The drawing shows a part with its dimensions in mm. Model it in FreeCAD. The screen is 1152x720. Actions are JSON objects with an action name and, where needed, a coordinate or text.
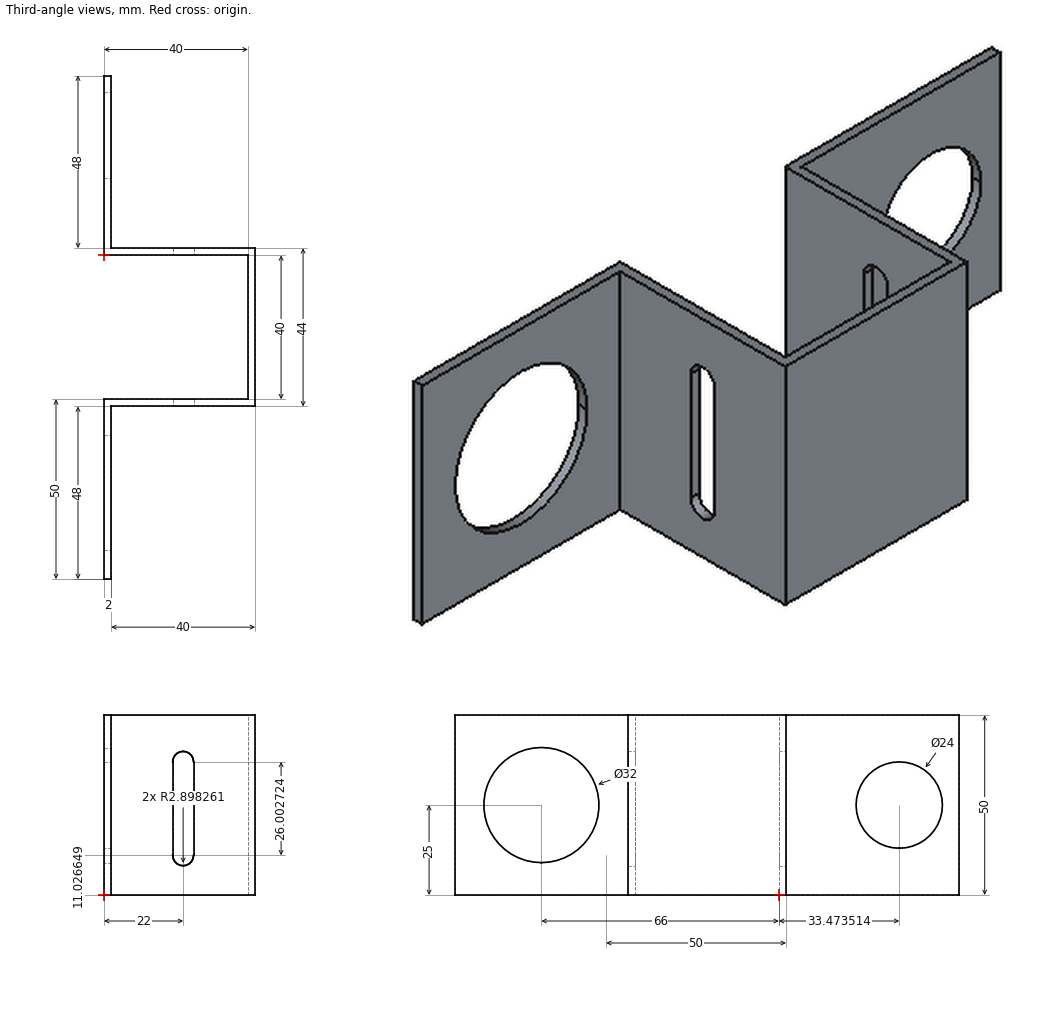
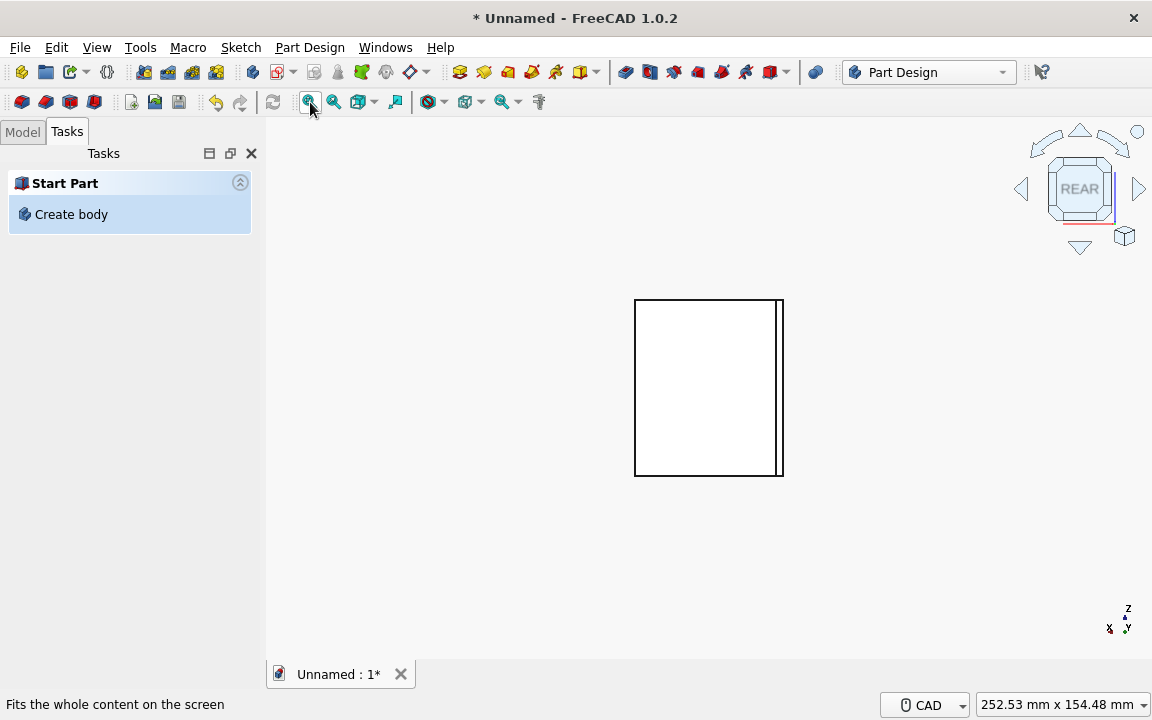
{"action": "left_click", "coordinate": [310, 102]}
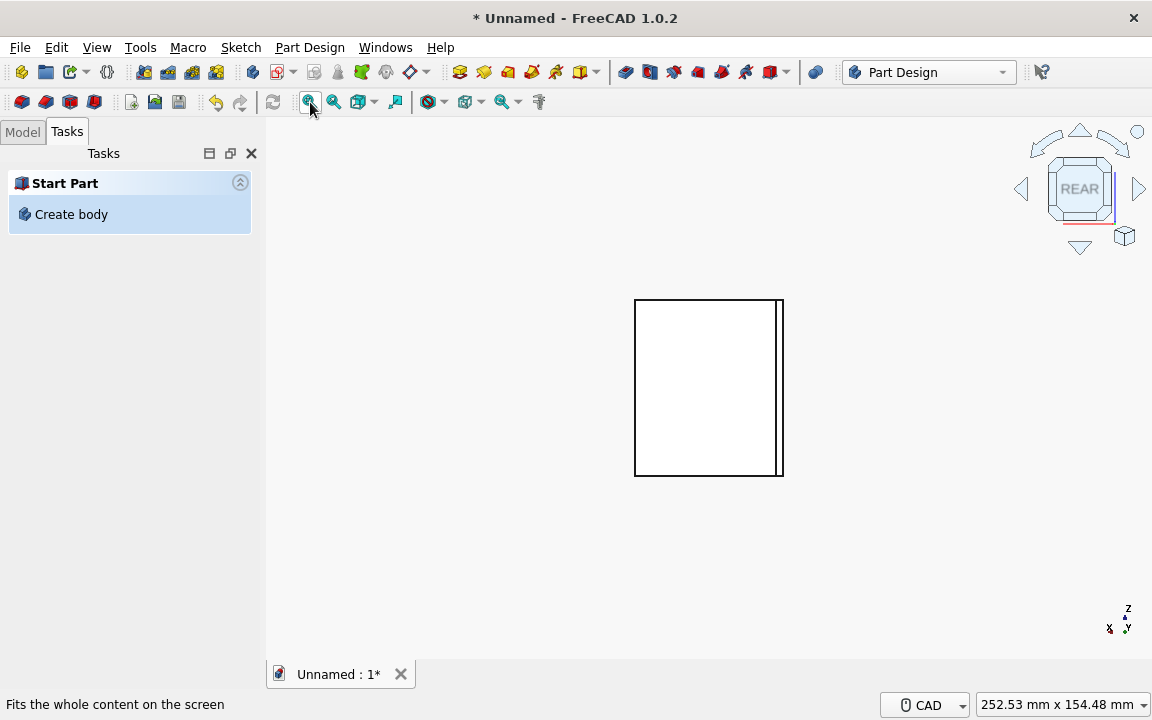
{"action": "left_click", "coordinate": [705, 387]}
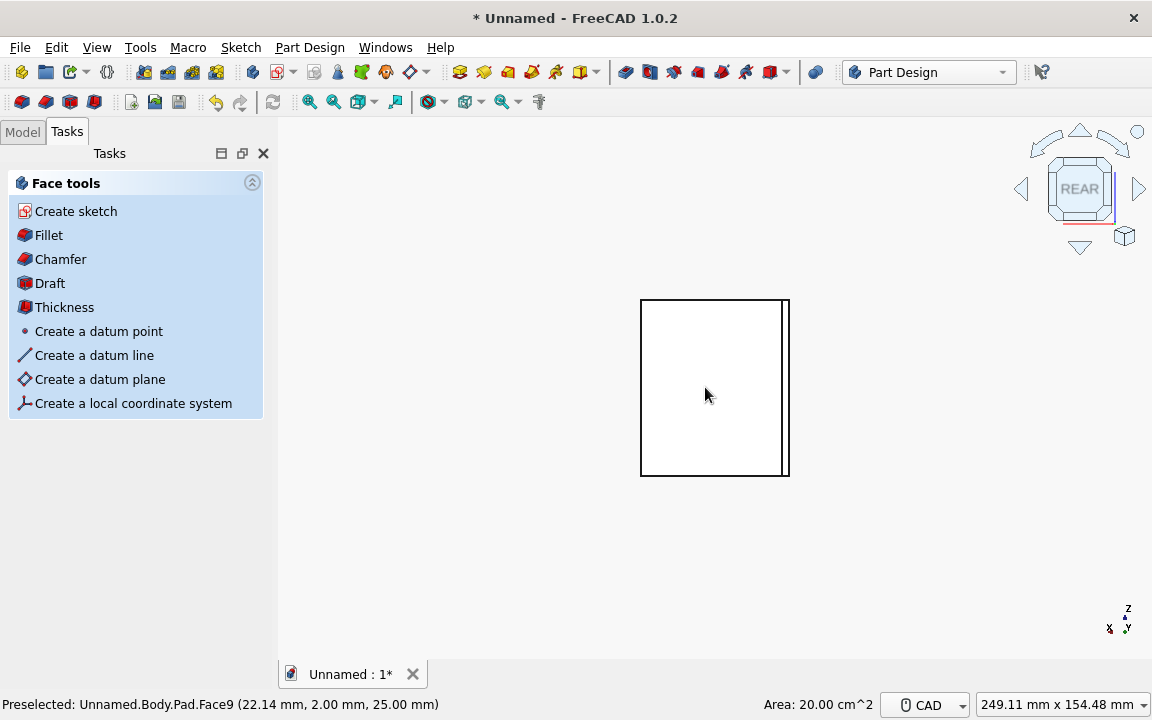
{"action": "left_click", "coordinate": [278, 72]}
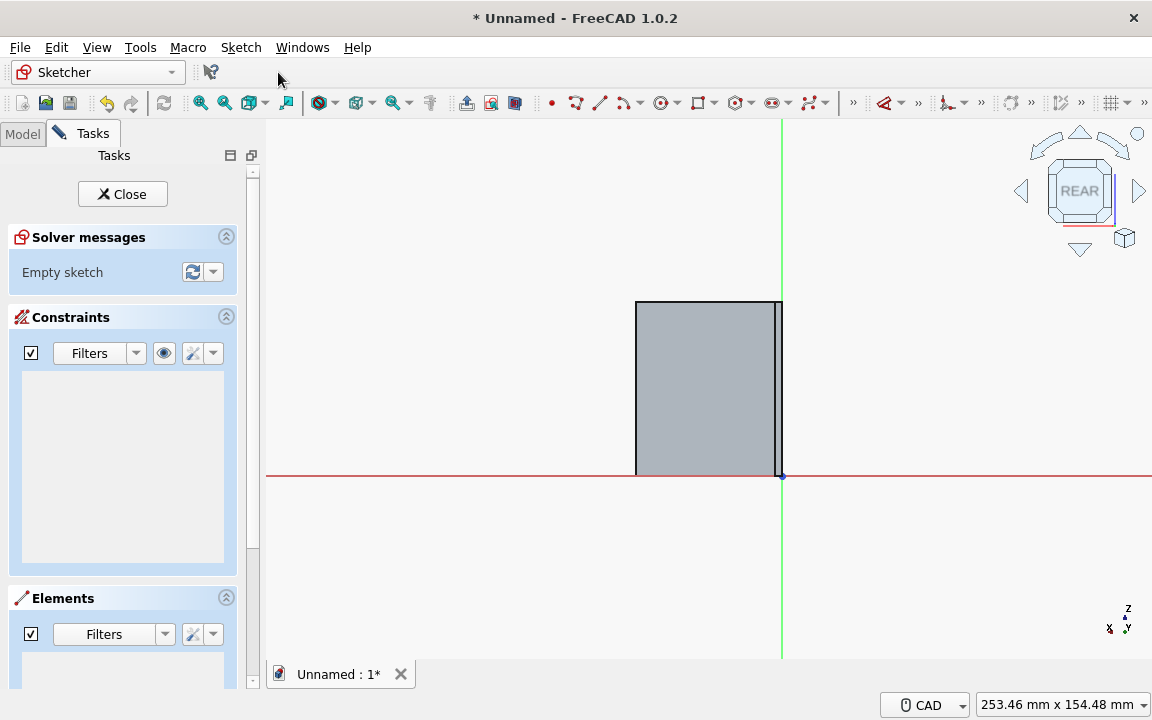
{"action": "left_click", "coordinate": [516, 104]}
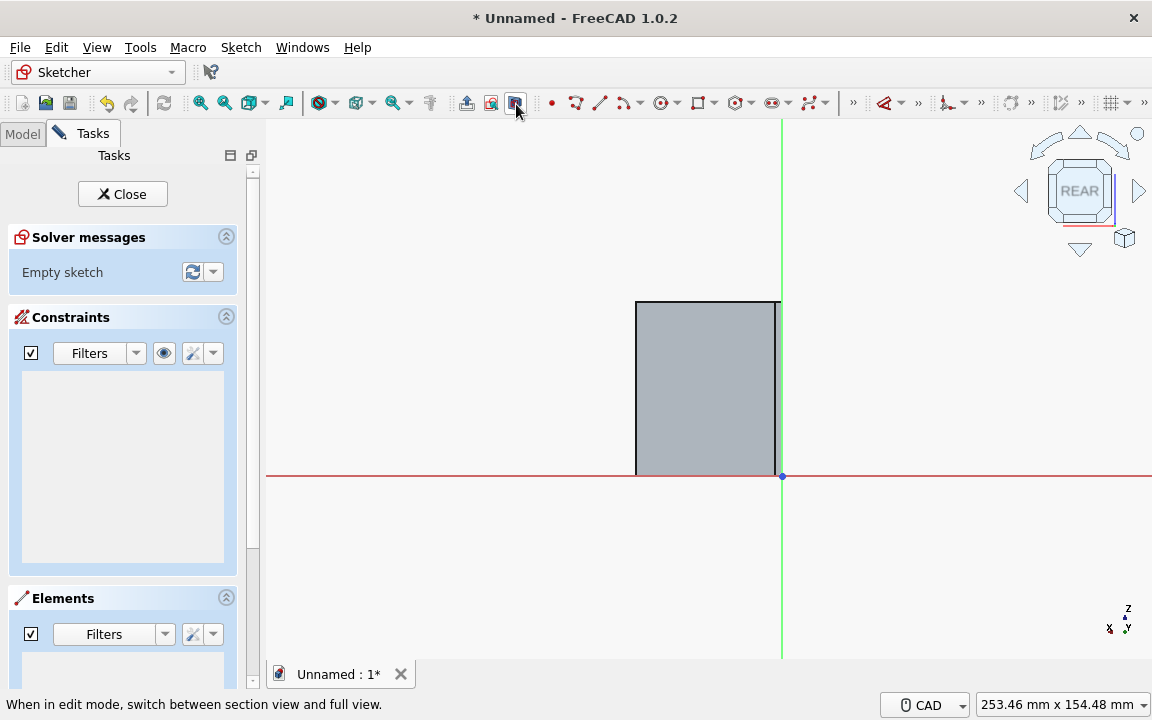
{"action": "scroll", "coordinate": [819, 421], "scroll_direction": "up", "scroll_amount": 4}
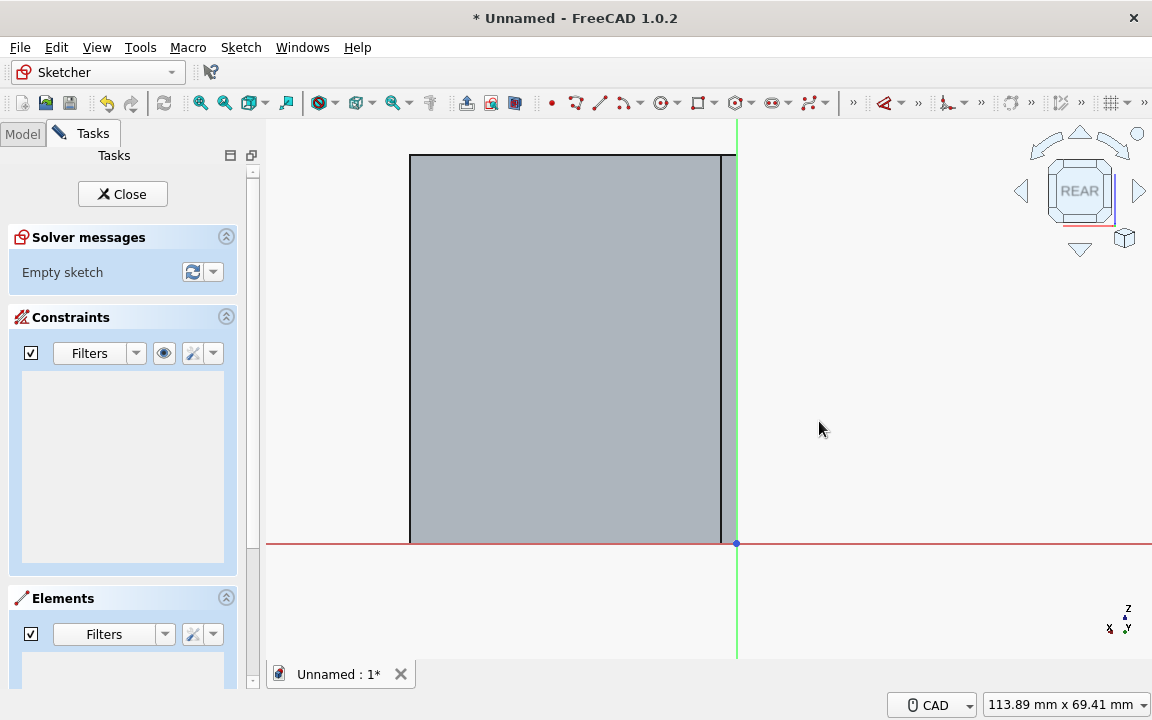
{"action": "left_click", "coordinate": [772, 104]}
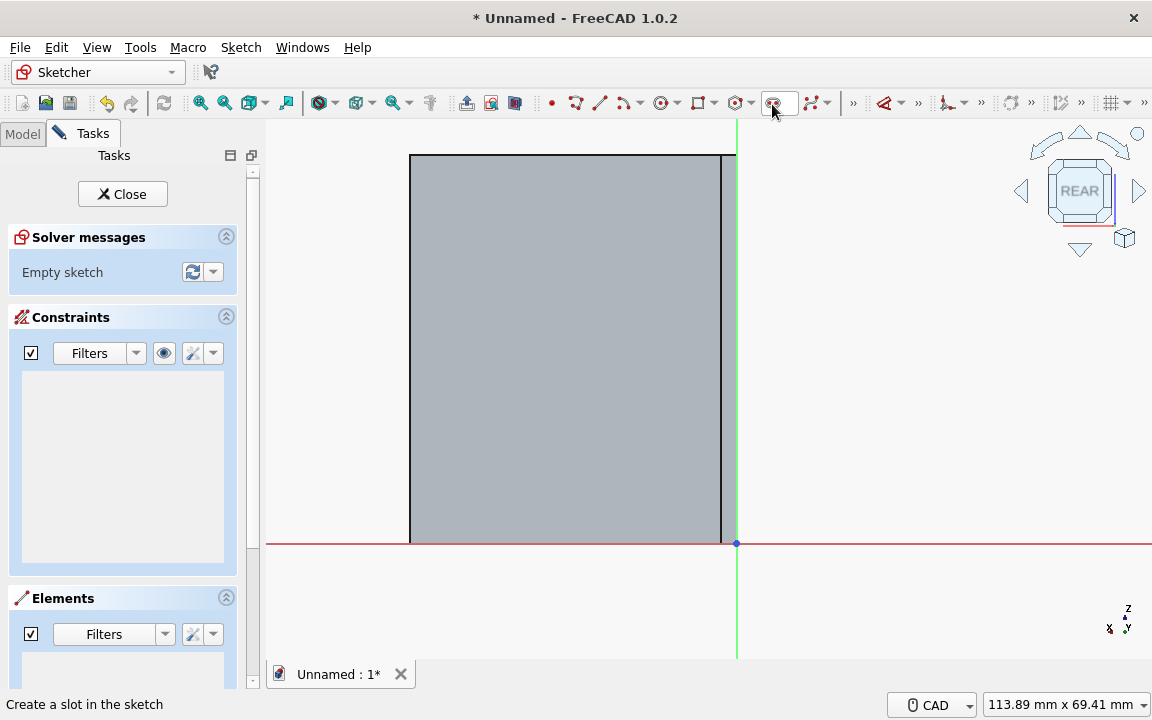
{"action": "left_click", "coordinate": [566, 458]}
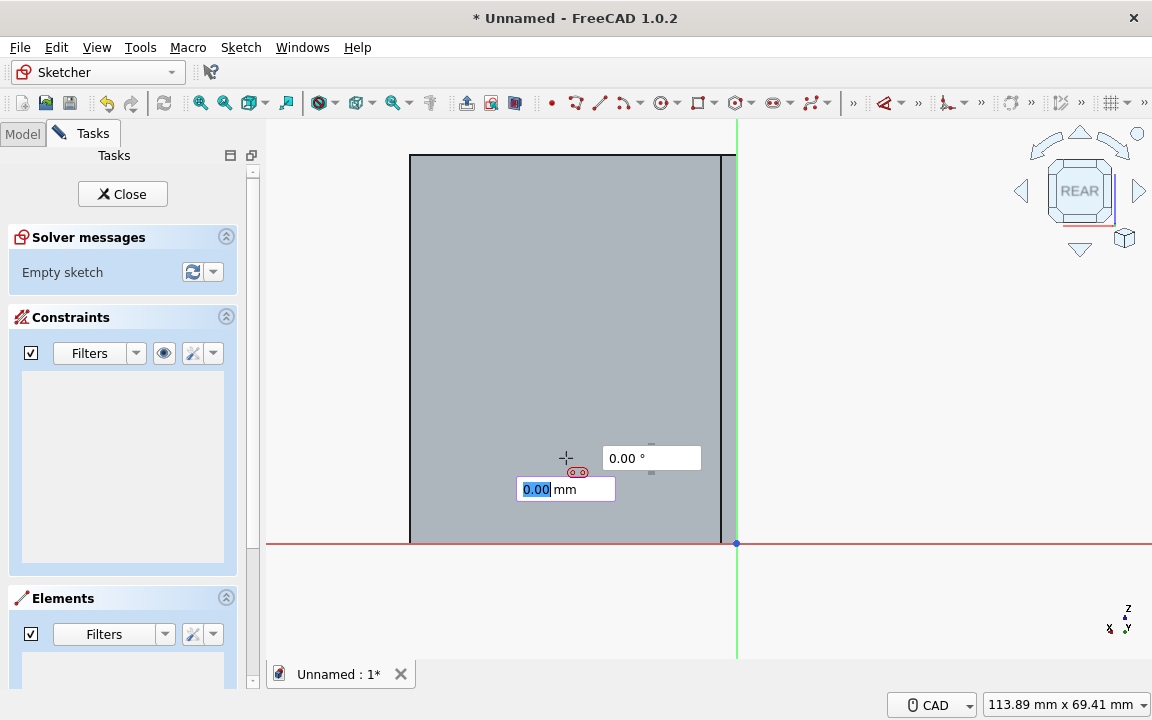
{"action": "left_click", "coordinate": [566, 256]}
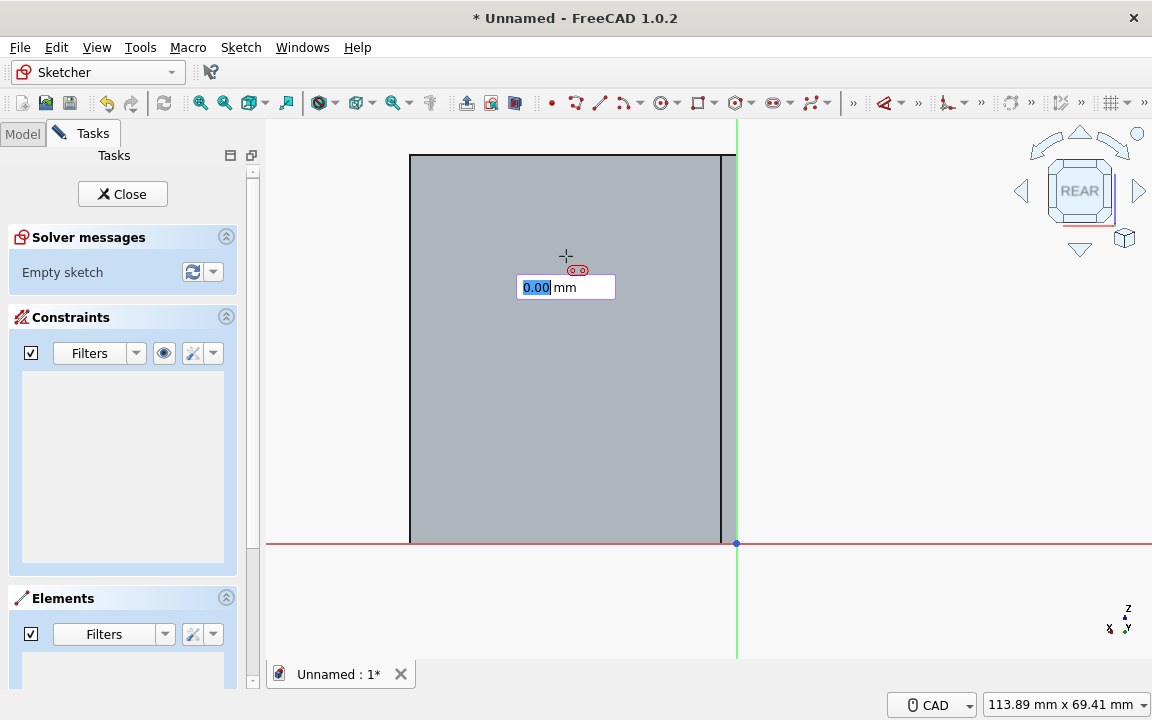
{"action": "left_click", "coordinate": [543, 357]}
{"action": "key", "text": "Escape"}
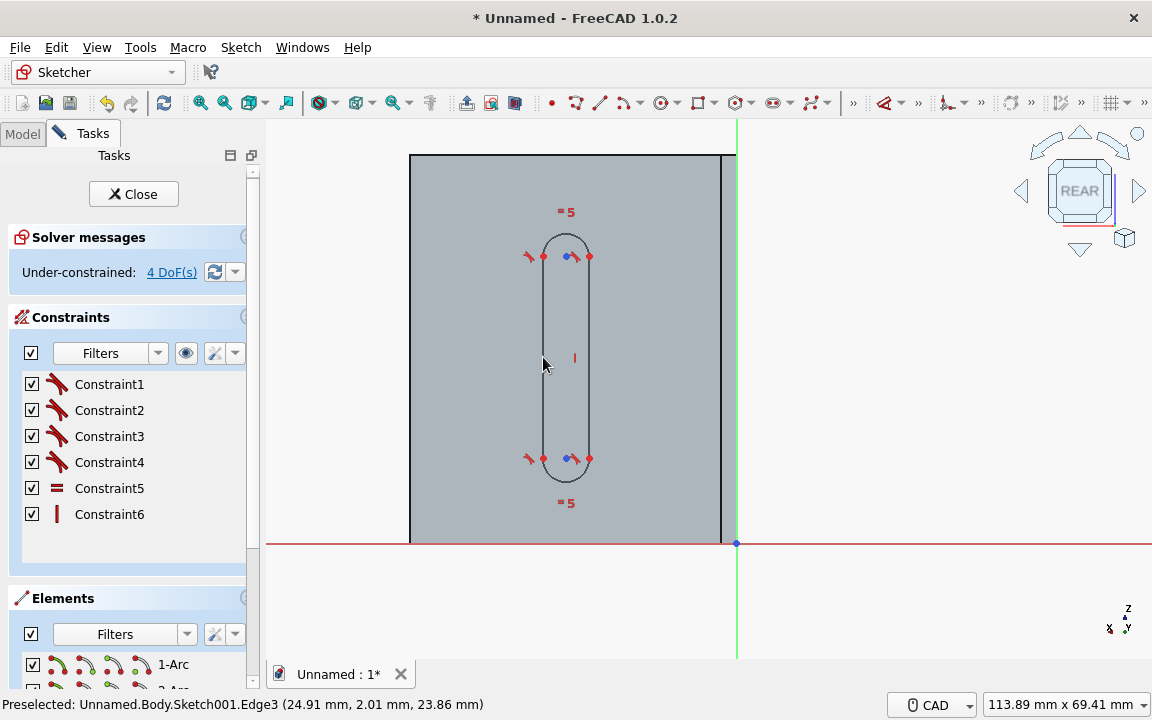
{"action": "left_click", "coordinate": [884, 104]}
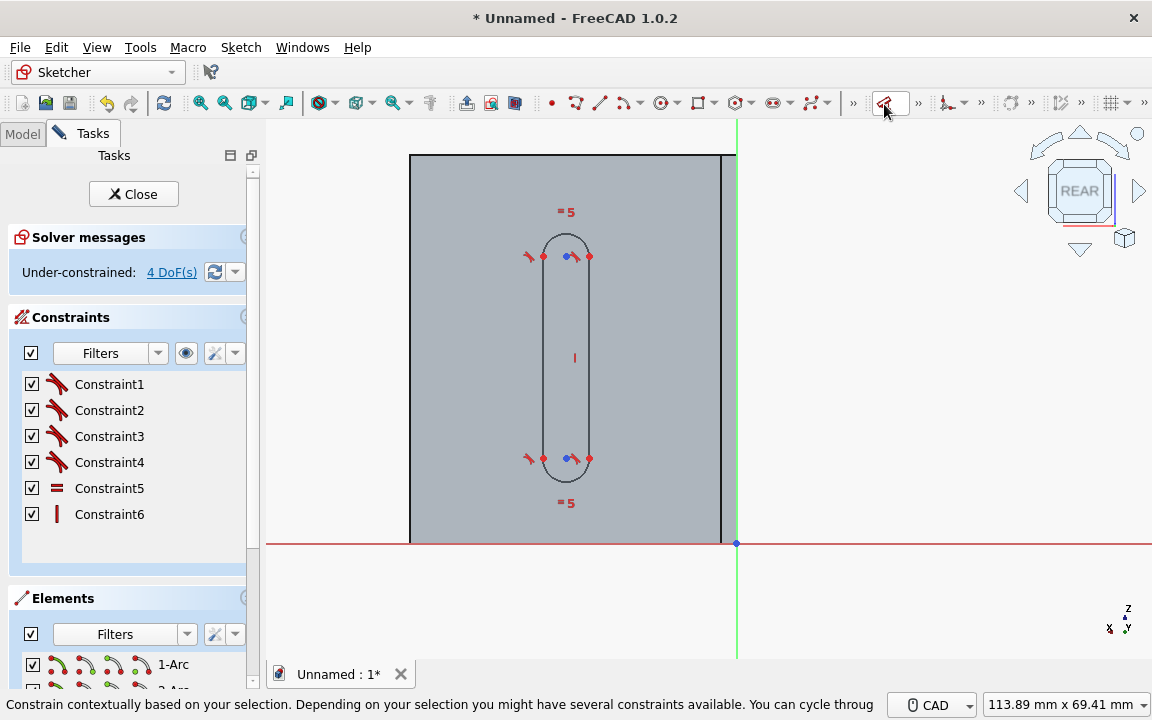
{"action": "scroll", "coordinate": [552, 478], "scroll_direction": "up", "scroll_amount": 3}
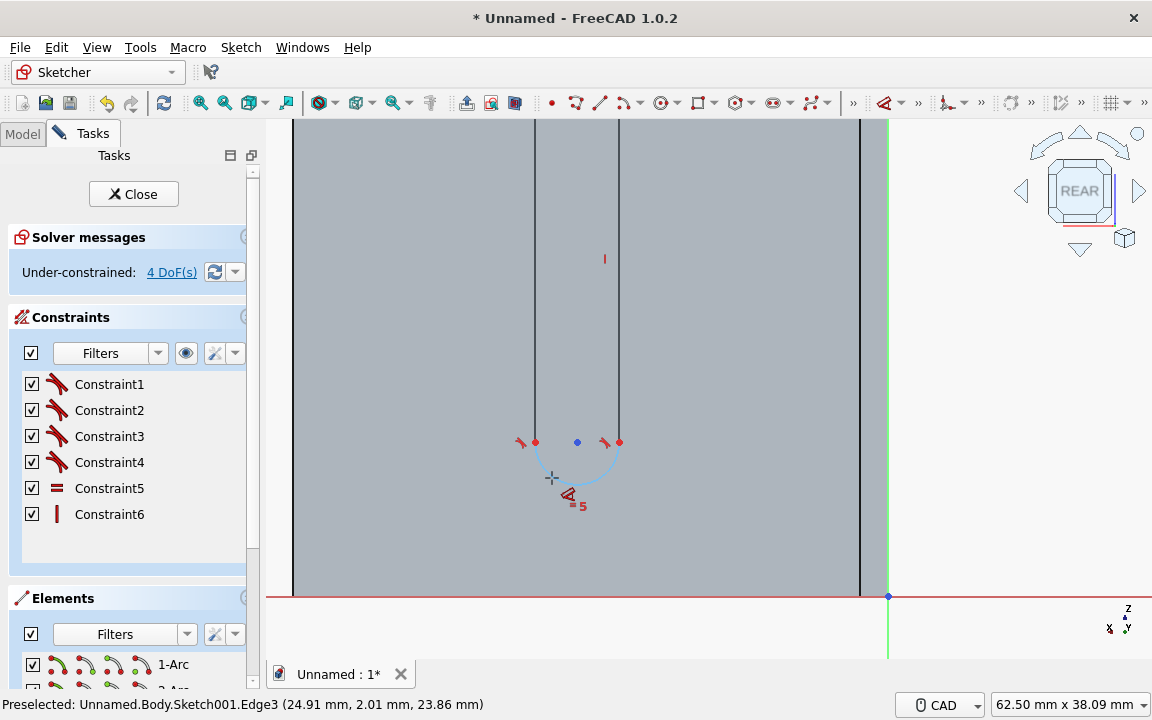
{"action": "left_click", "coordinate": [553, 477]}
{"action": "left_click", "coordinate": [534, 503]}